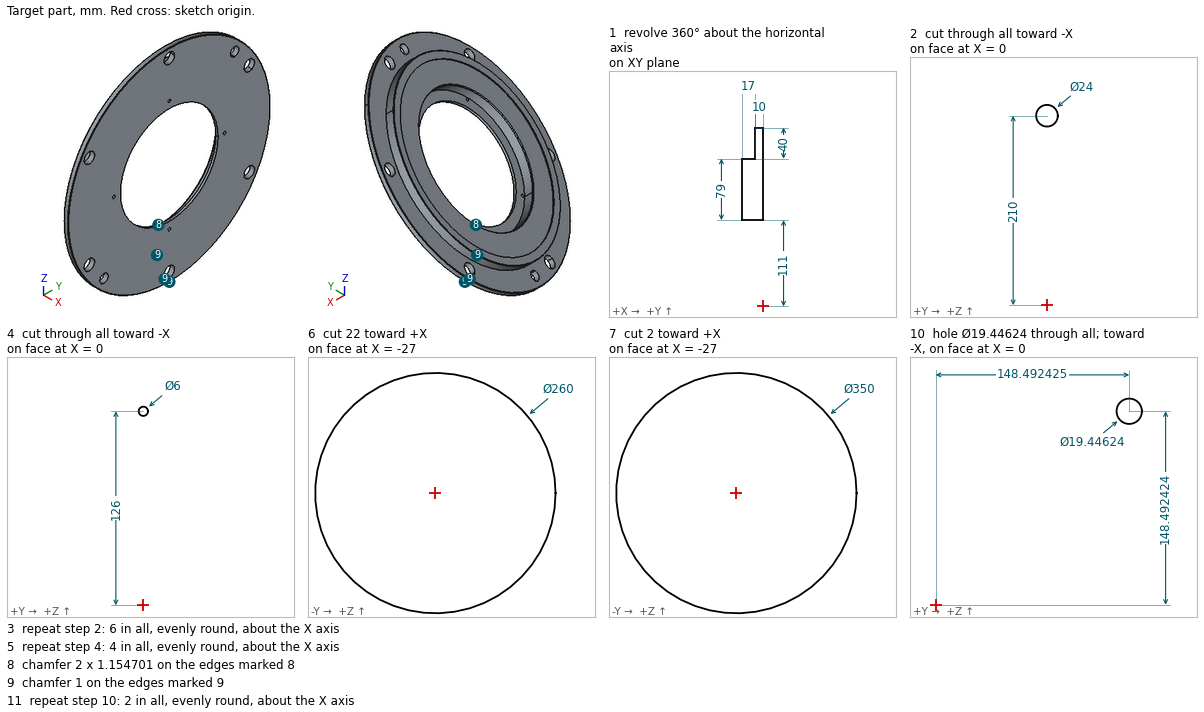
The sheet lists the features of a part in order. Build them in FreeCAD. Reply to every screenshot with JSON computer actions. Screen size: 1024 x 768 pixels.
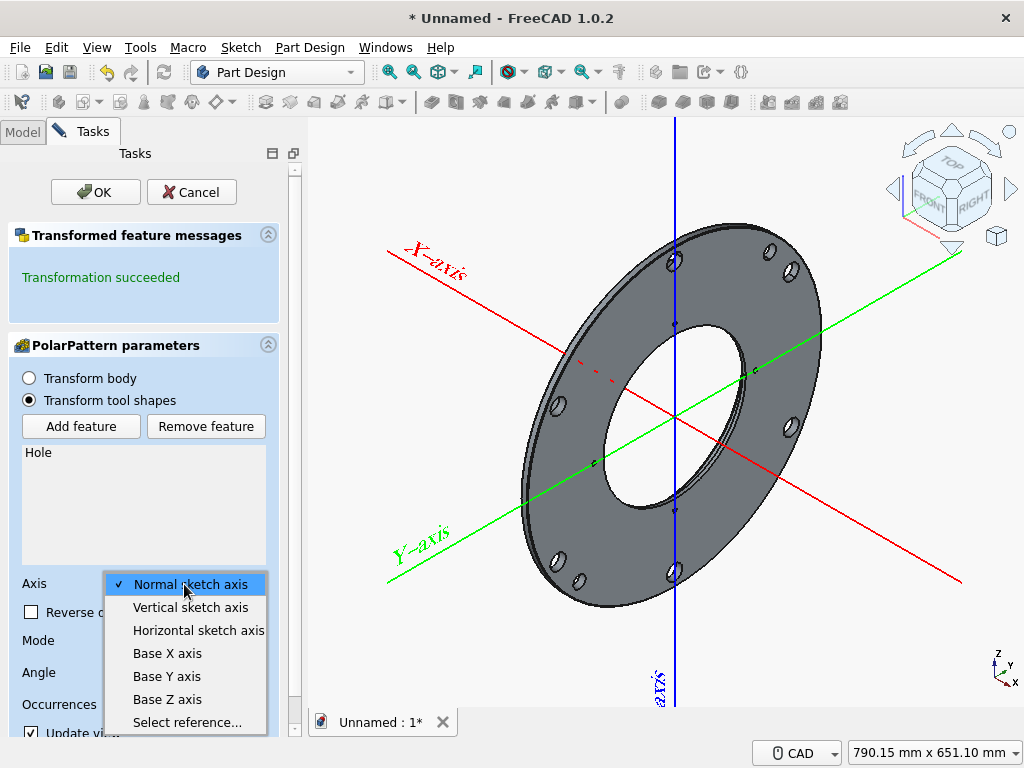
{"action": "left_click", "coordinate": [184, 654]}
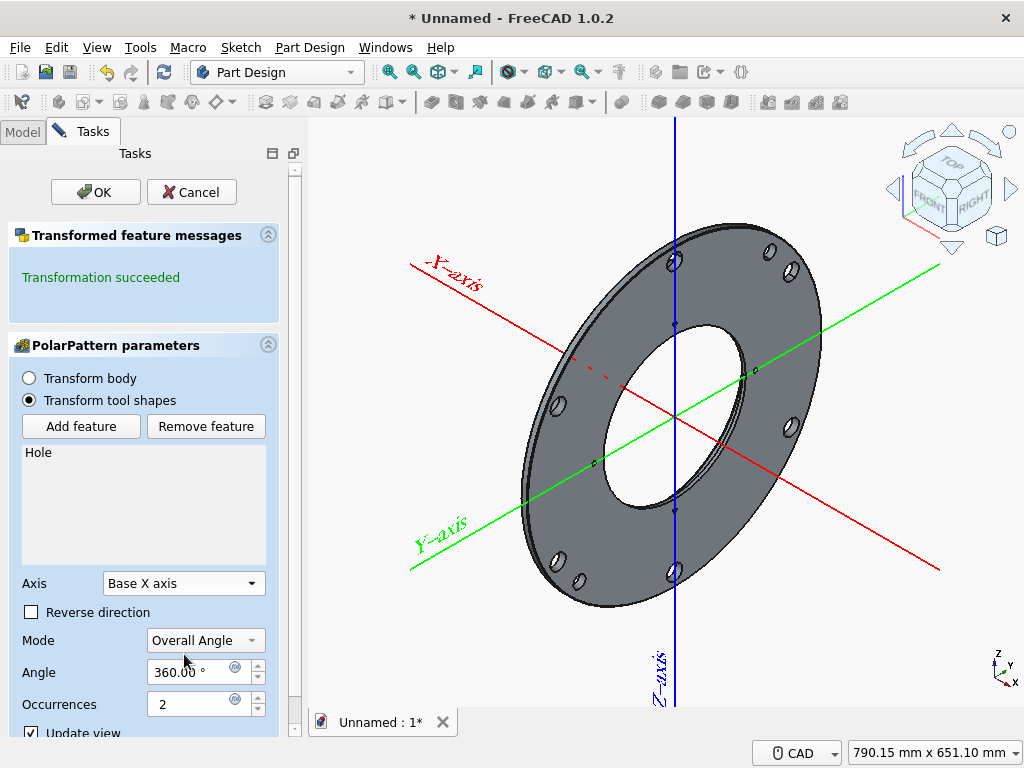
{"action": "triple_click", "coordinate": [198, 704]}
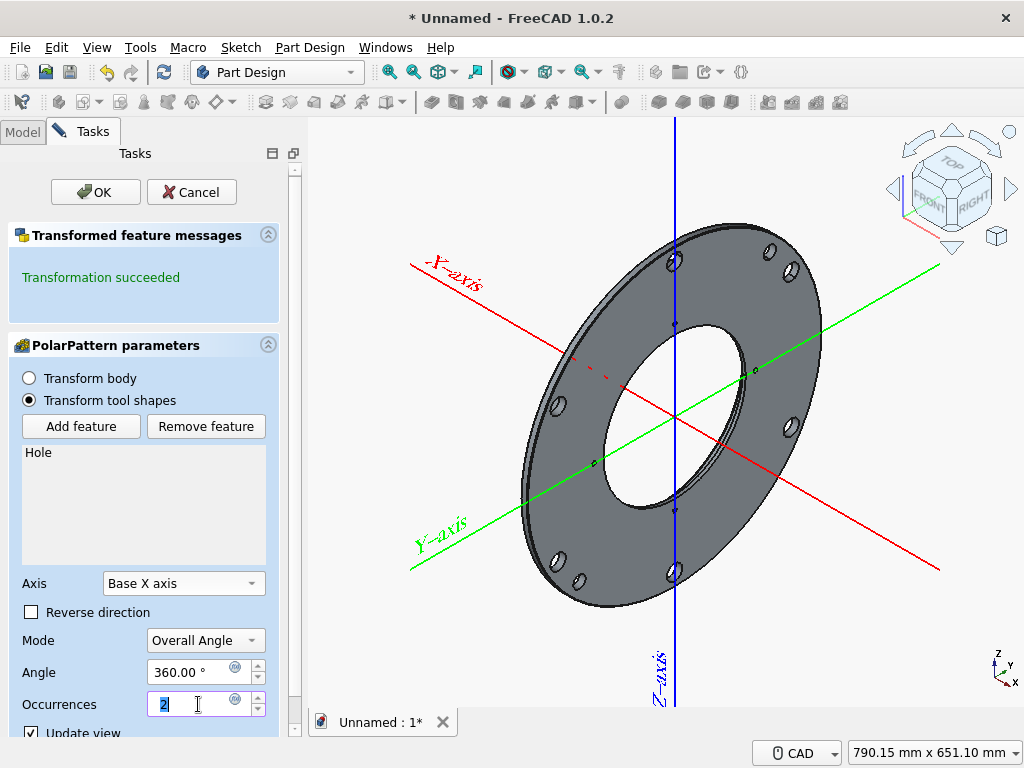
{"action": "type", "text": "2"}
{"action": "key", "text": "Tab"}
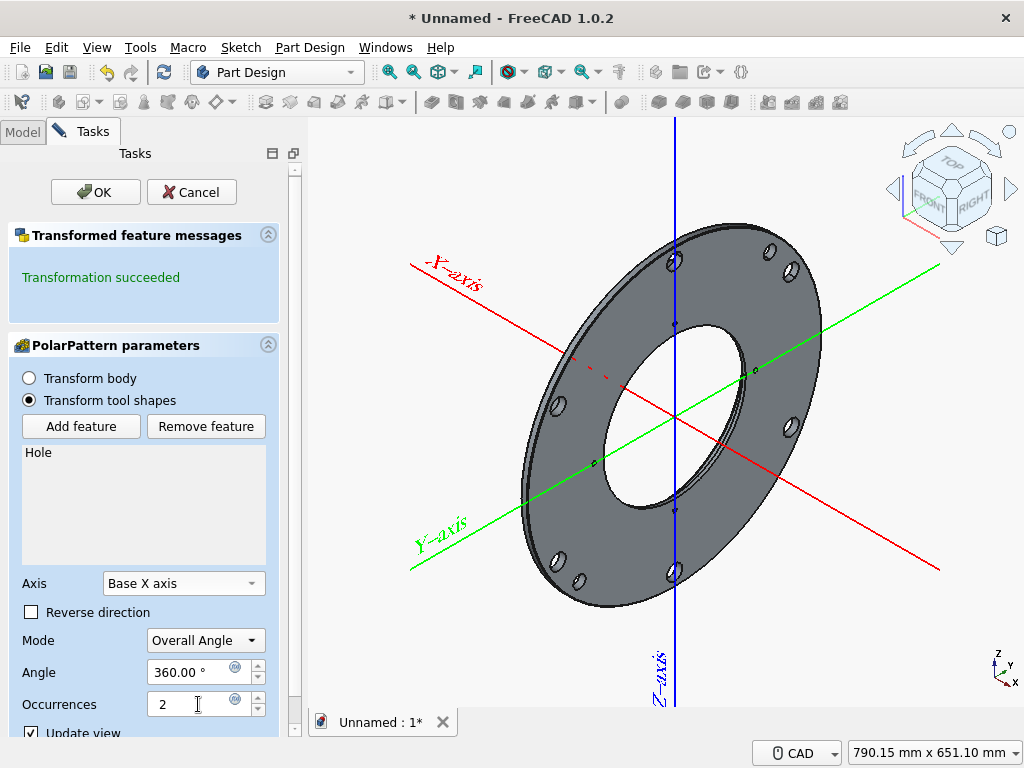
{"action": "left_click", "coordinate": [96, 192]}